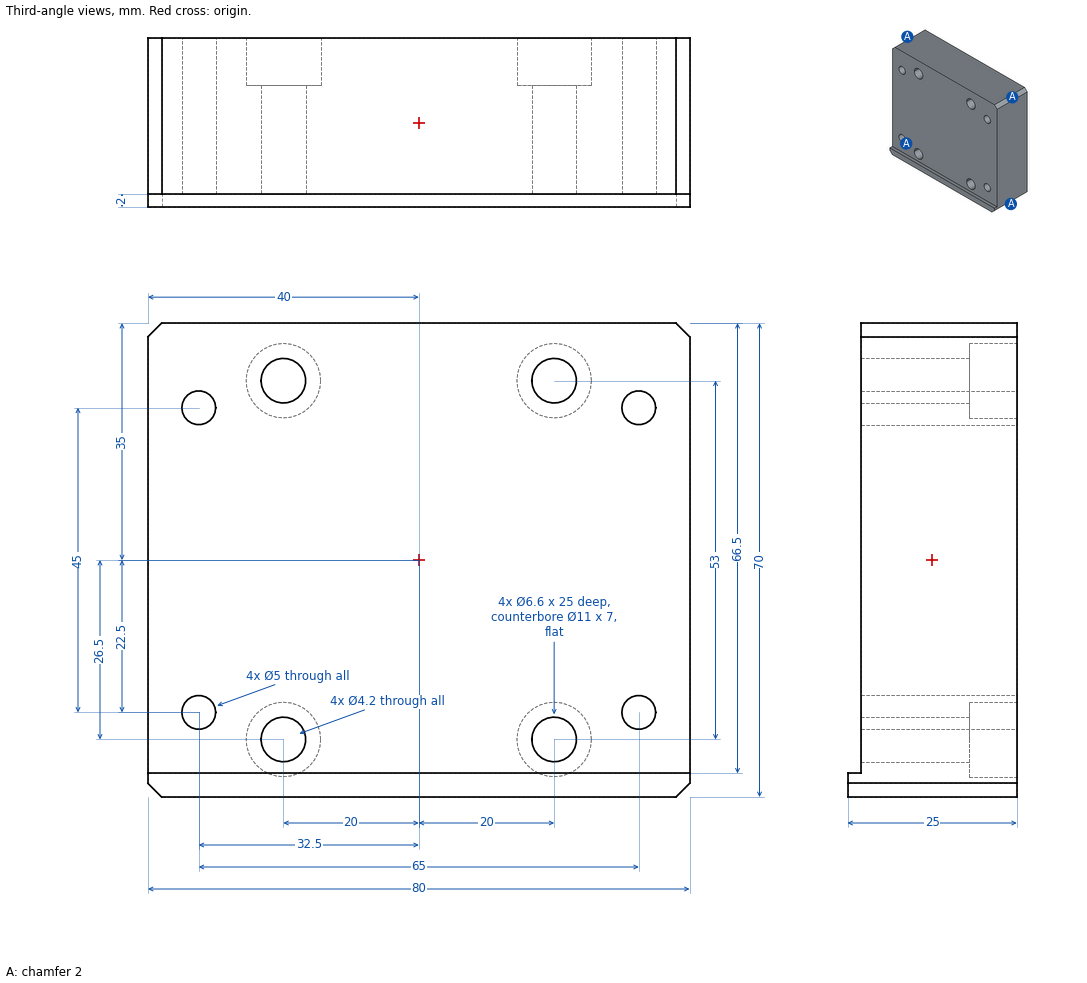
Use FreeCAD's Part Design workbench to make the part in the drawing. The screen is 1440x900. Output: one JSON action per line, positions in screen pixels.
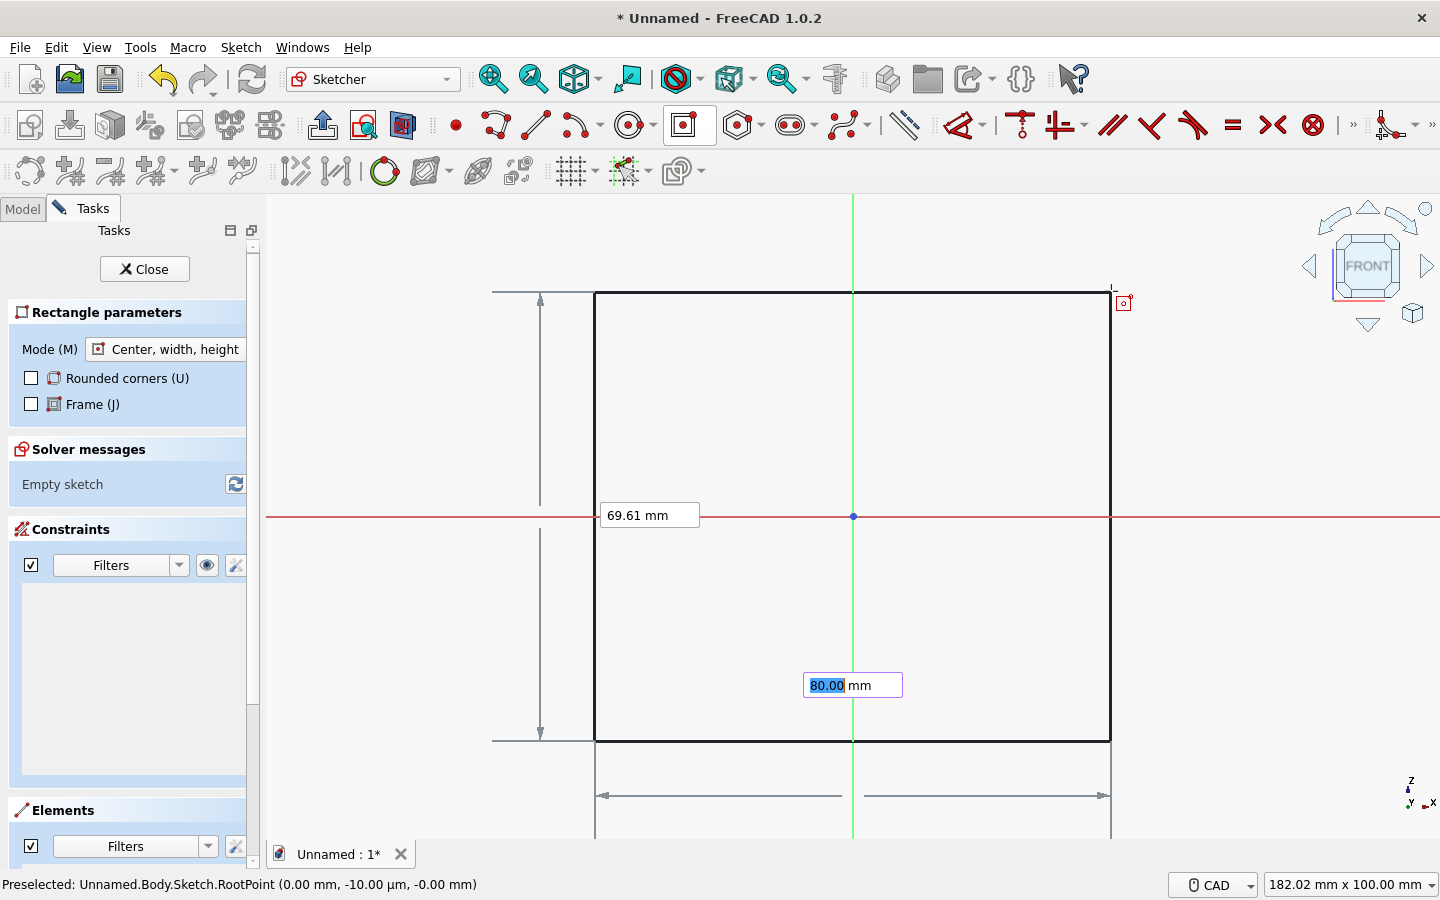
{"action": "type", "text": "80"}
{"action": "key", "text": "Tab"}
{"action": "type", "text": "70"}
{"action": "key", "text": "Return"}
{"action": "key", "text": "Escape"}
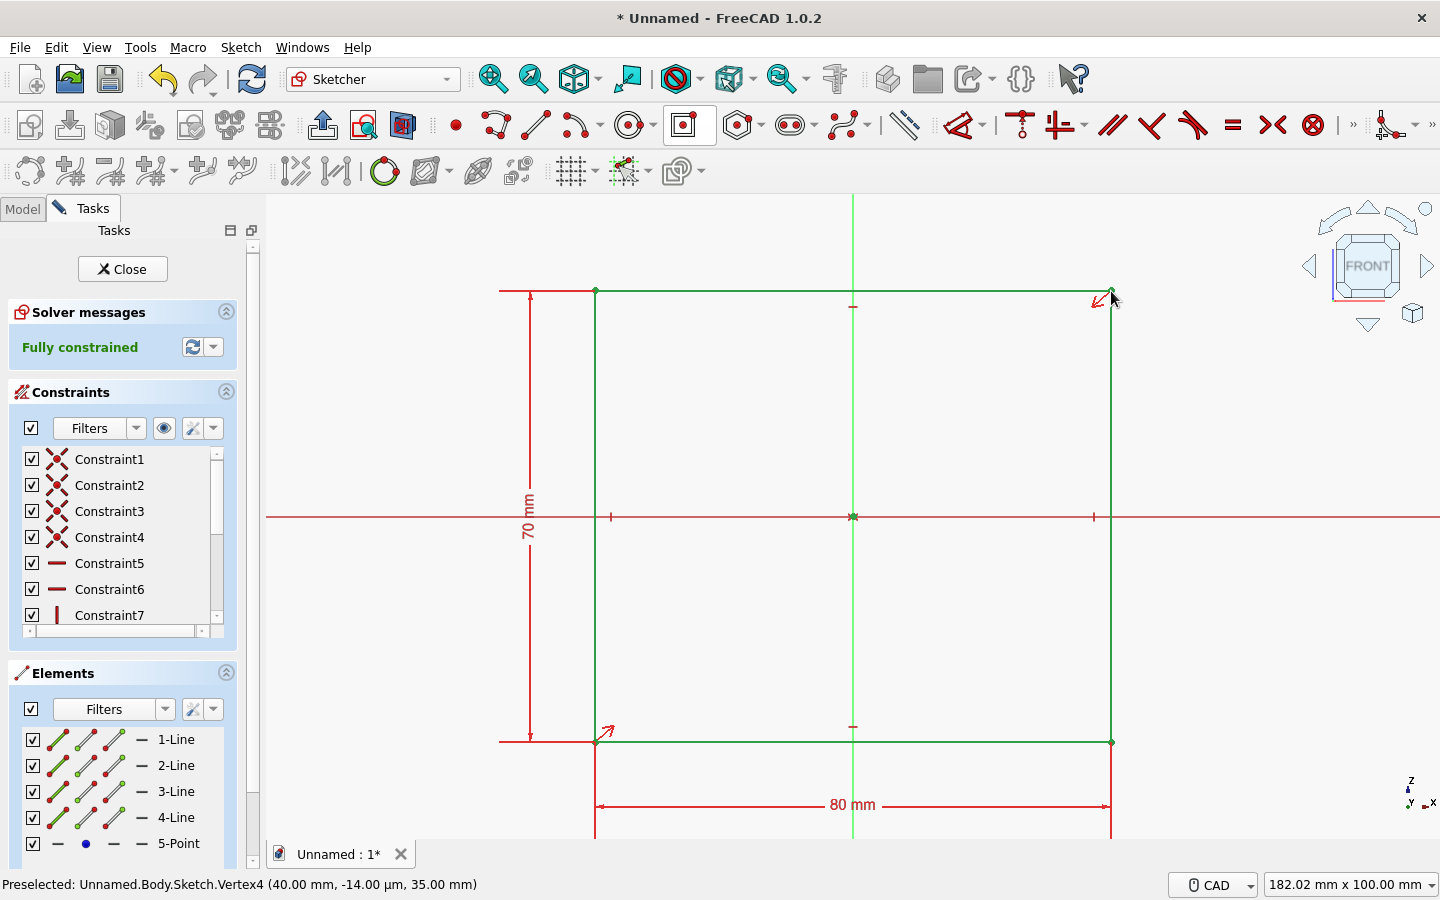
{"action": "left_click", "coordinate": [123, 269]}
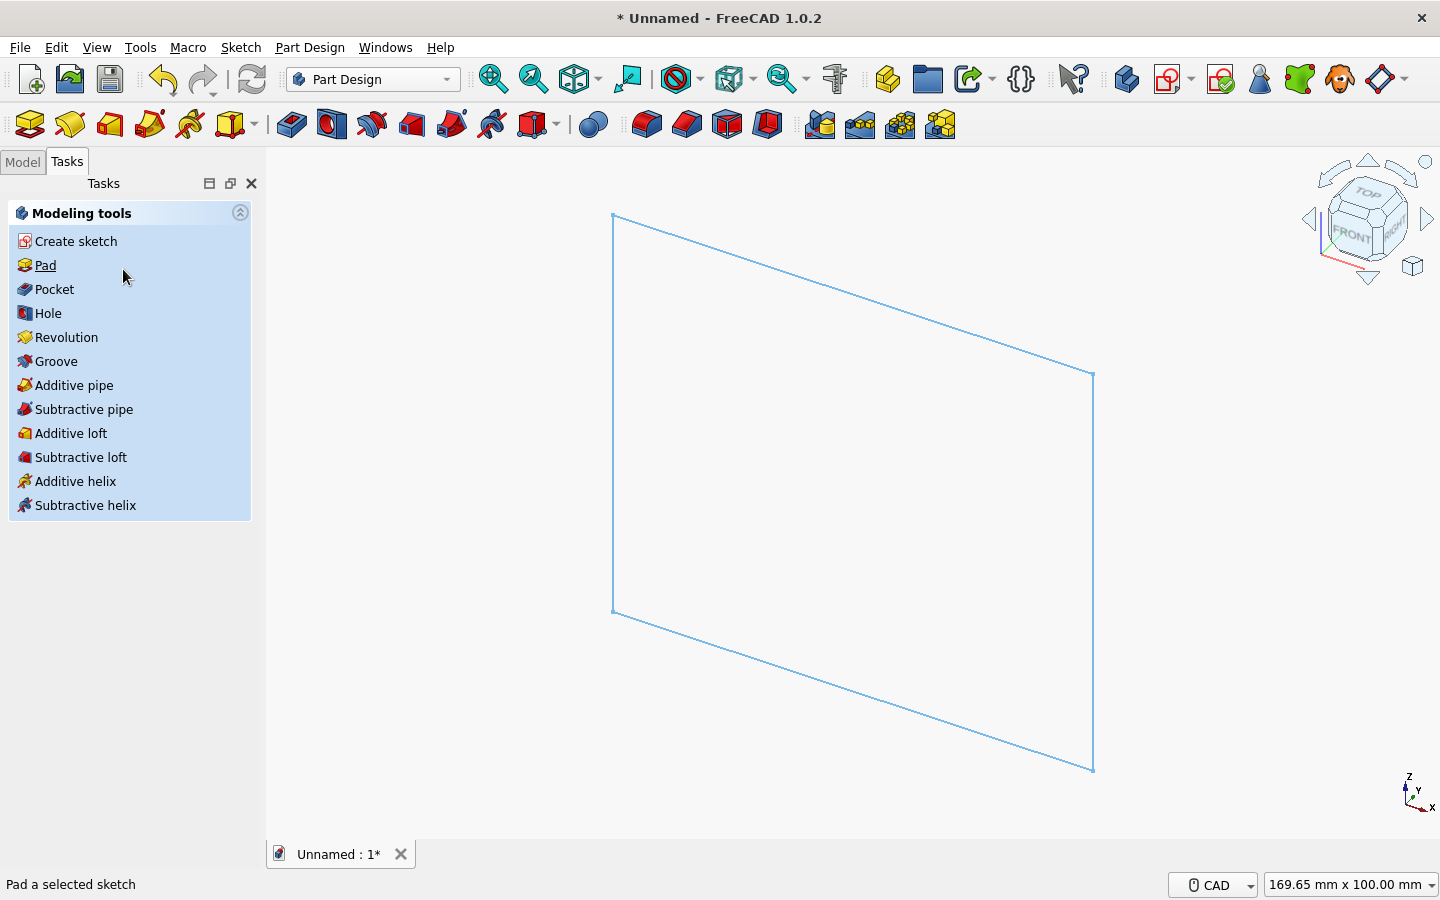
{"action": "left_click", "coordinate": [30, 124]}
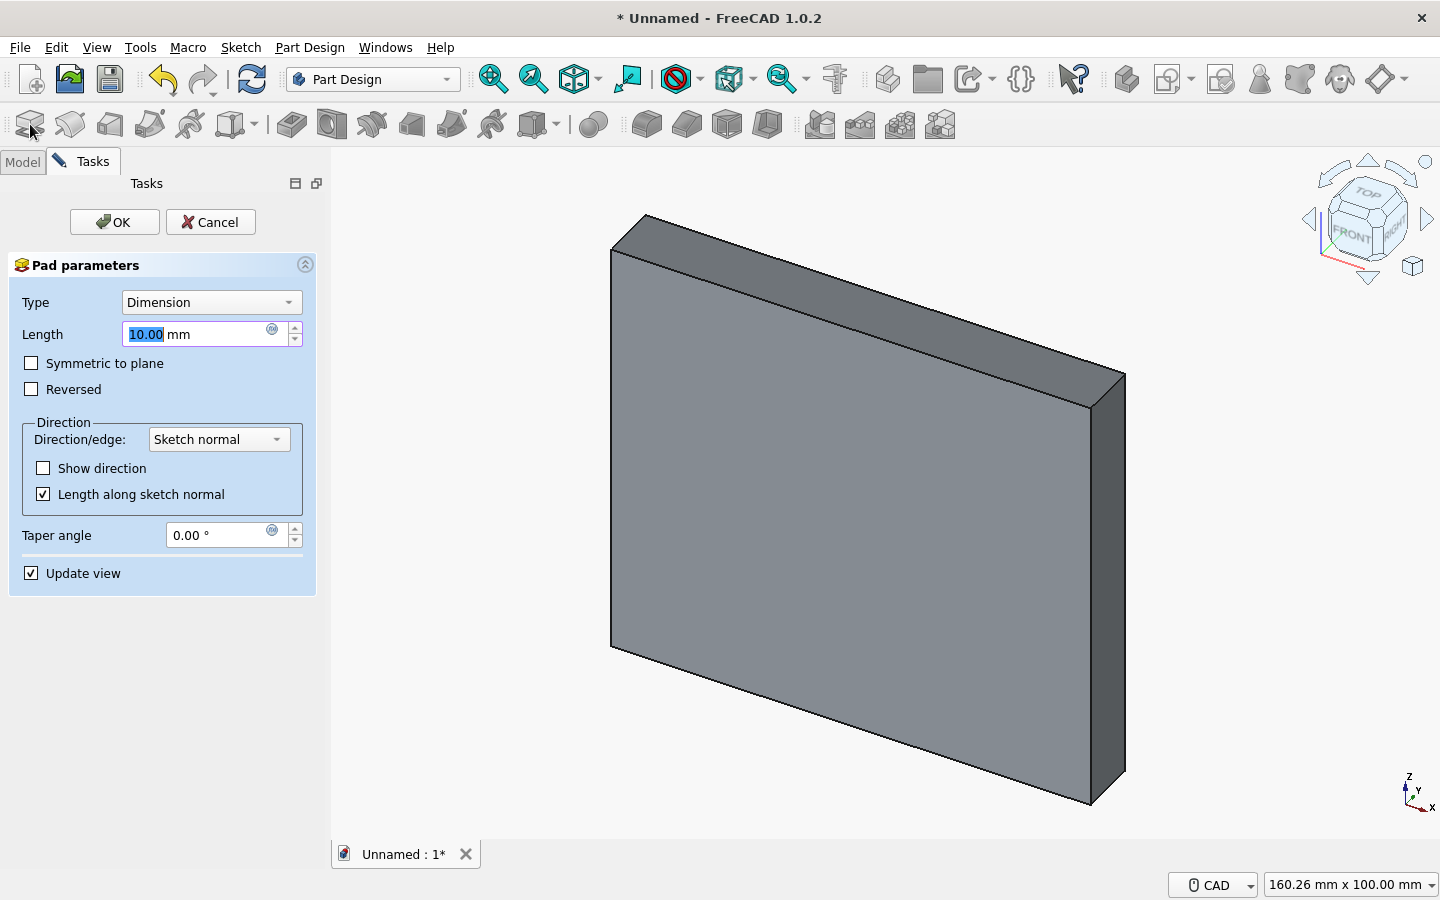
{"action": "type", "text": "25"}
{"action": "key", "text": "Tab"}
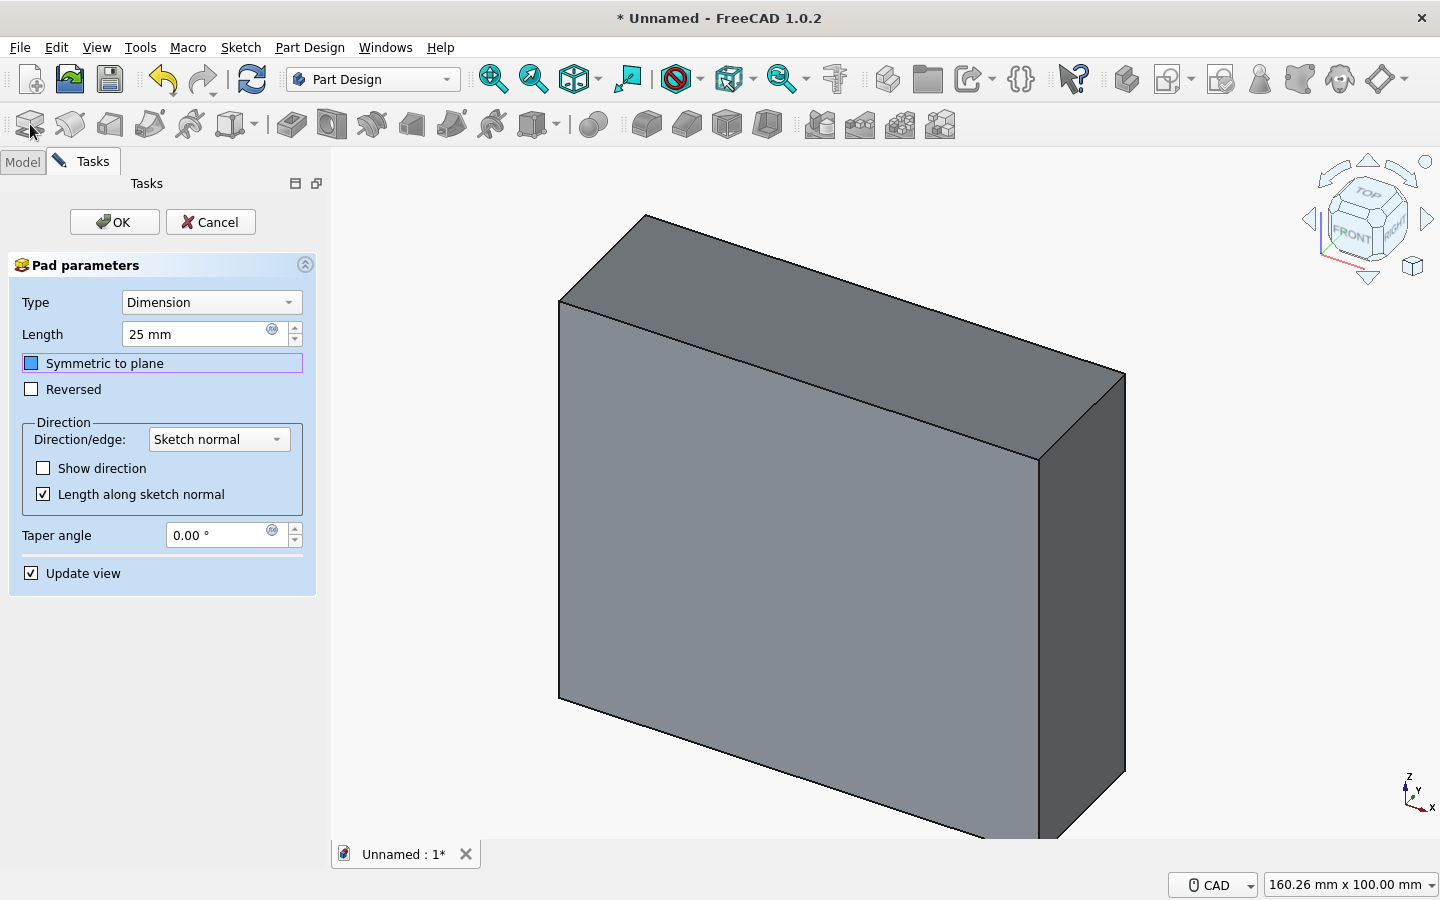
{"action": "left_click", "coordinate": [30, 363]}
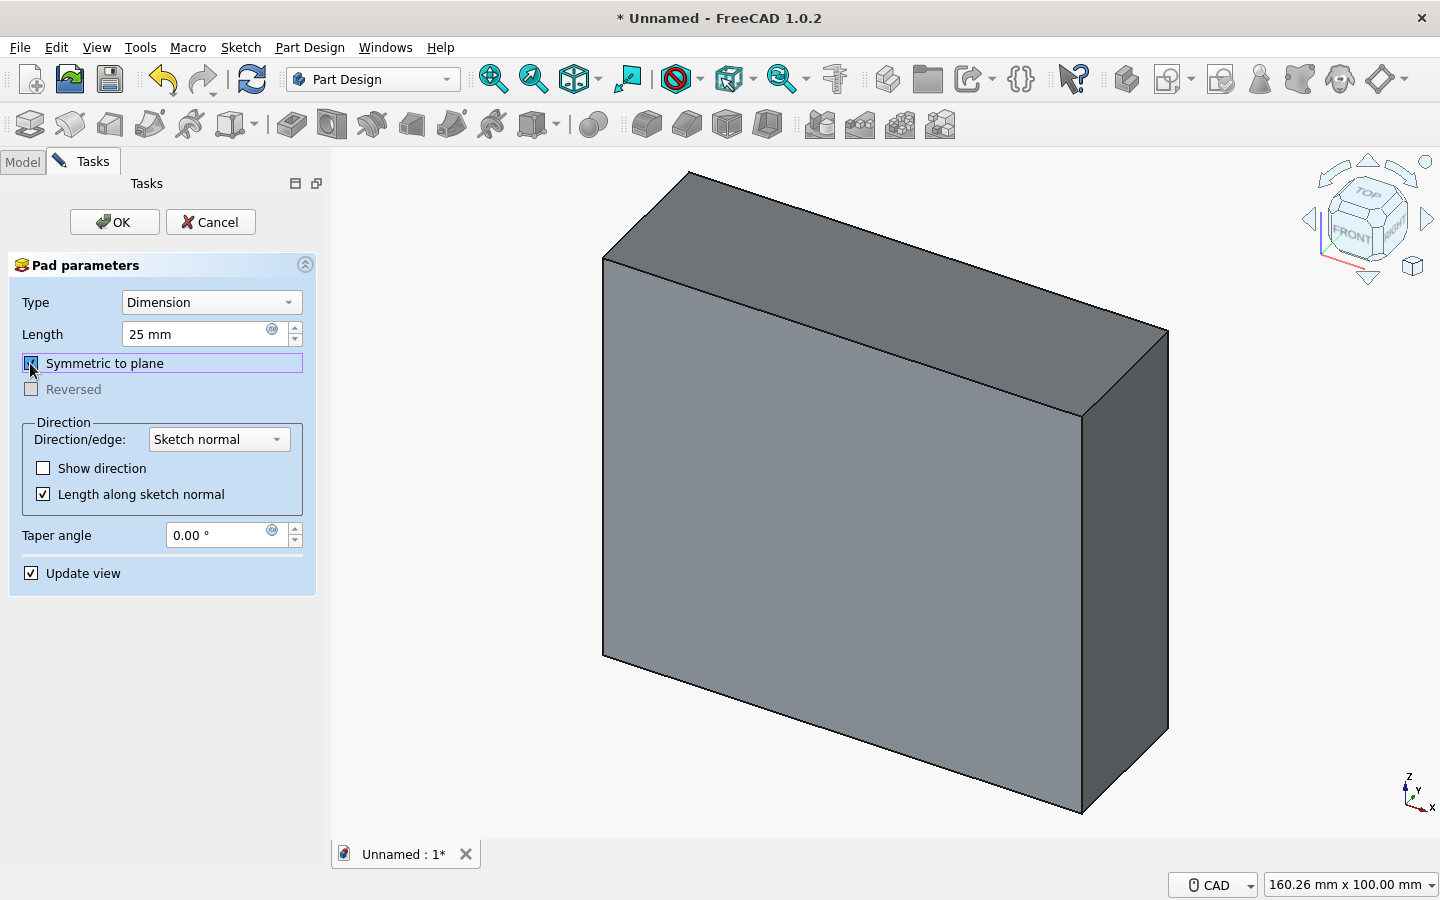
{"action": "left_click", "coordinate": [115, 222]}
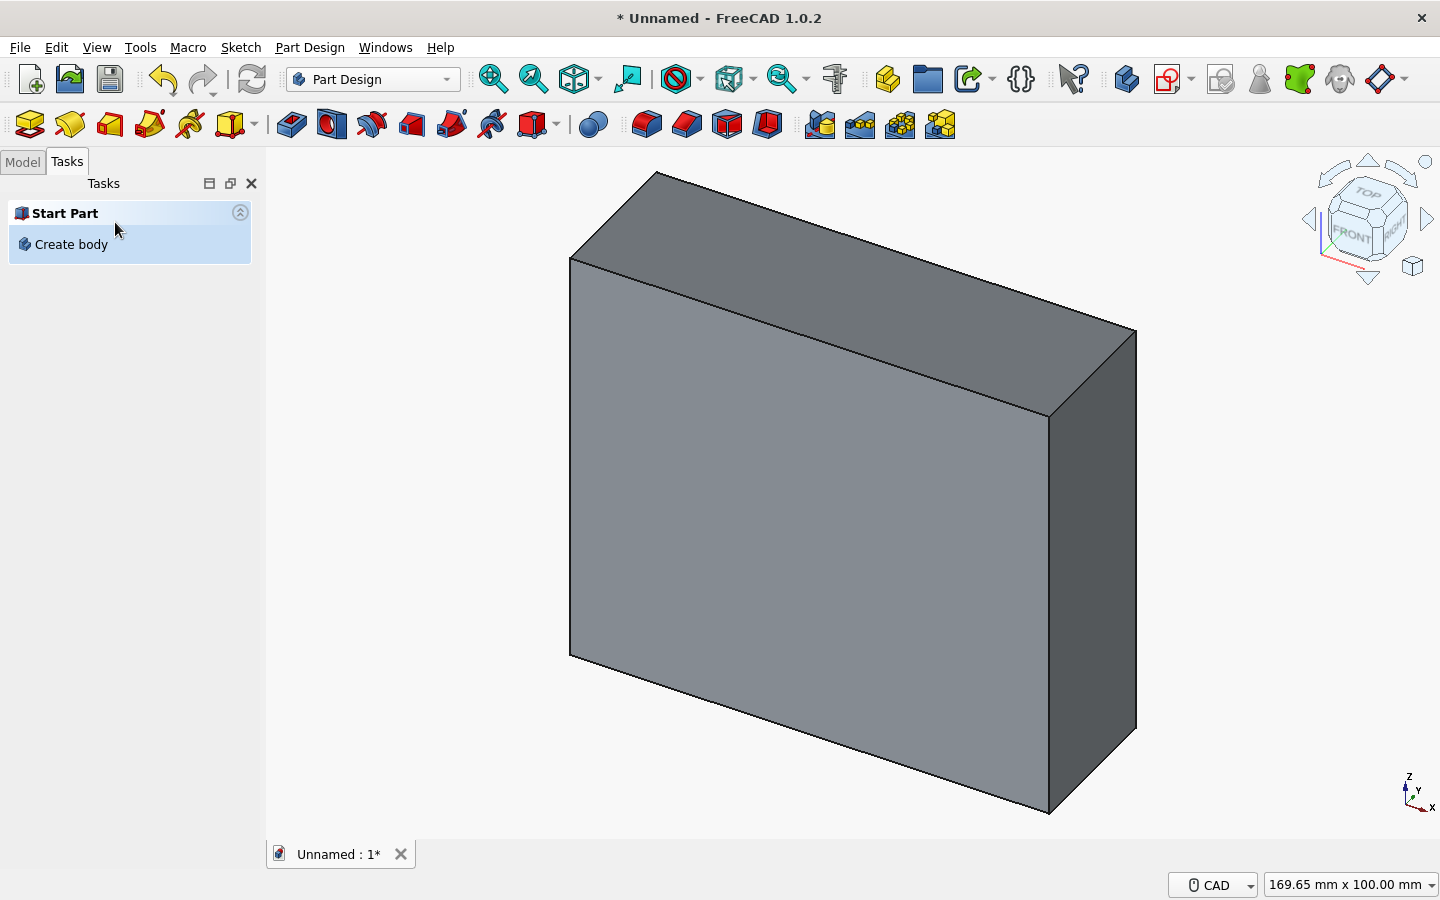
{"action": "left_click", "coordinate": [810, 535]}